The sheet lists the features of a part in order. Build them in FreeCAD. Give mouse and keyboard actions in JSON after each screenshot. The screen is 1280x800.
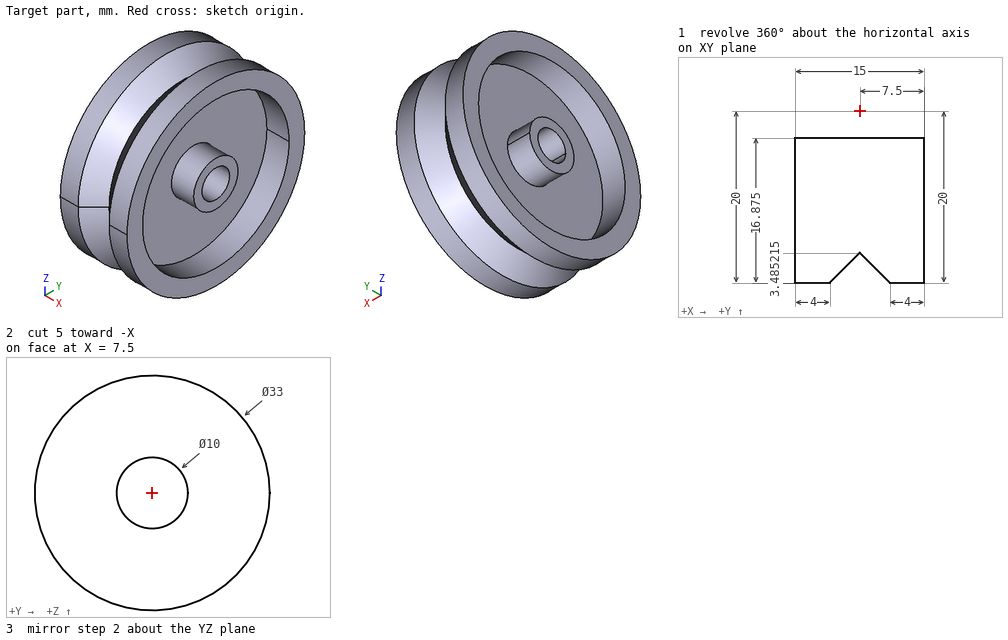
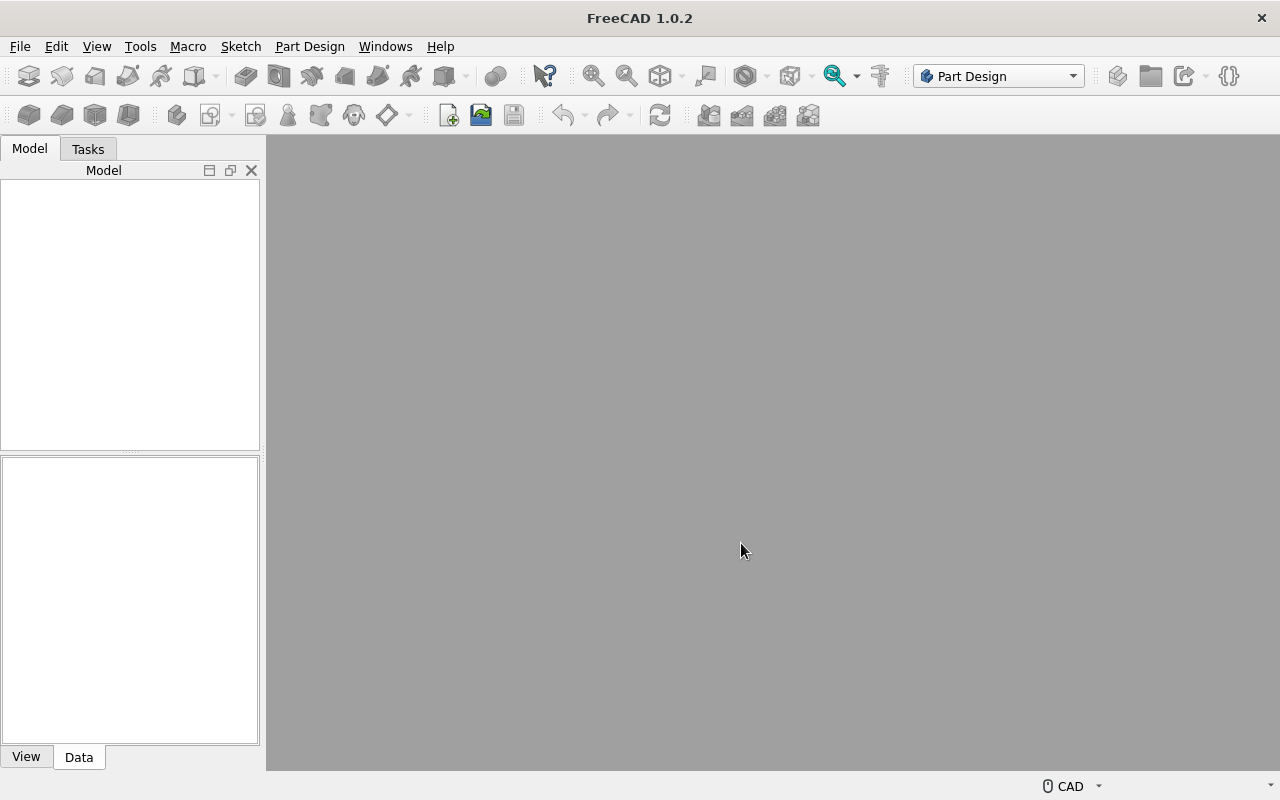
{"action": "left_click", "coordinate": [448, 116]}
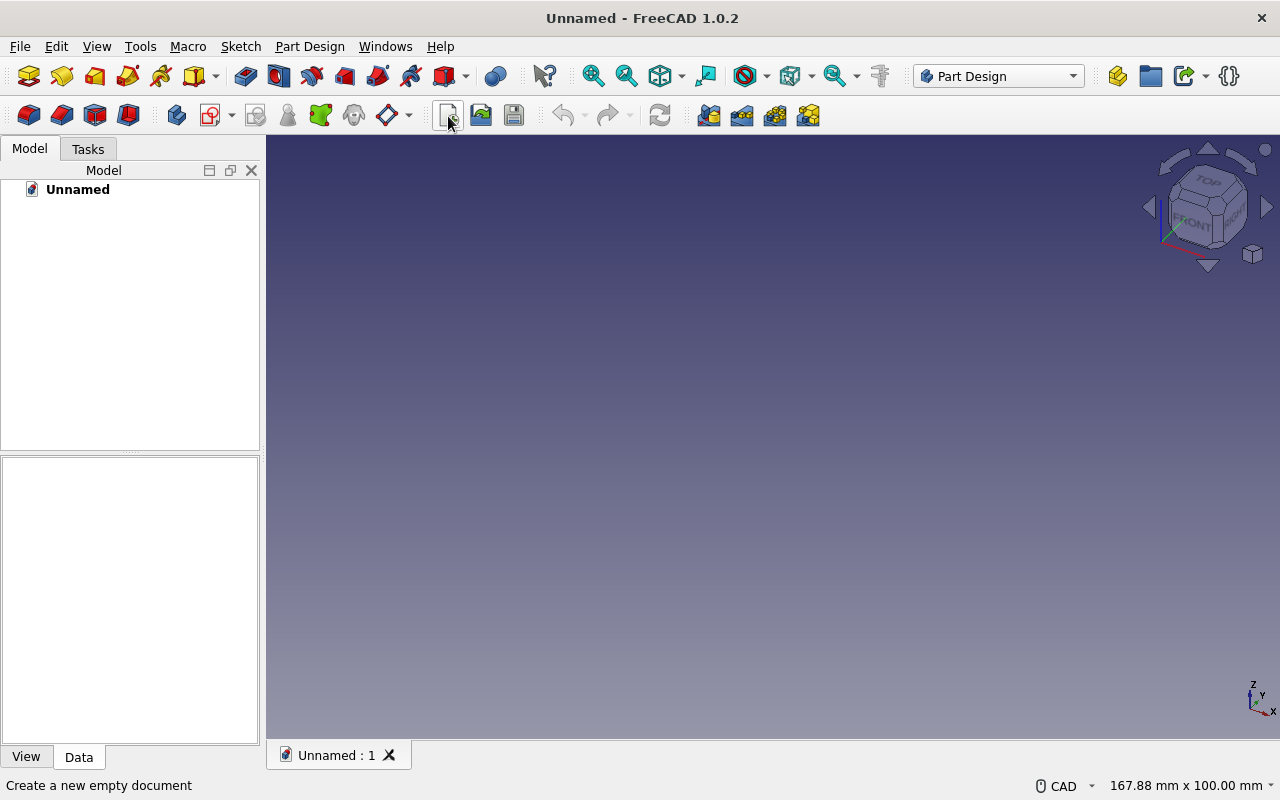
{"action": "left_click", "coordinate": [210, 116]}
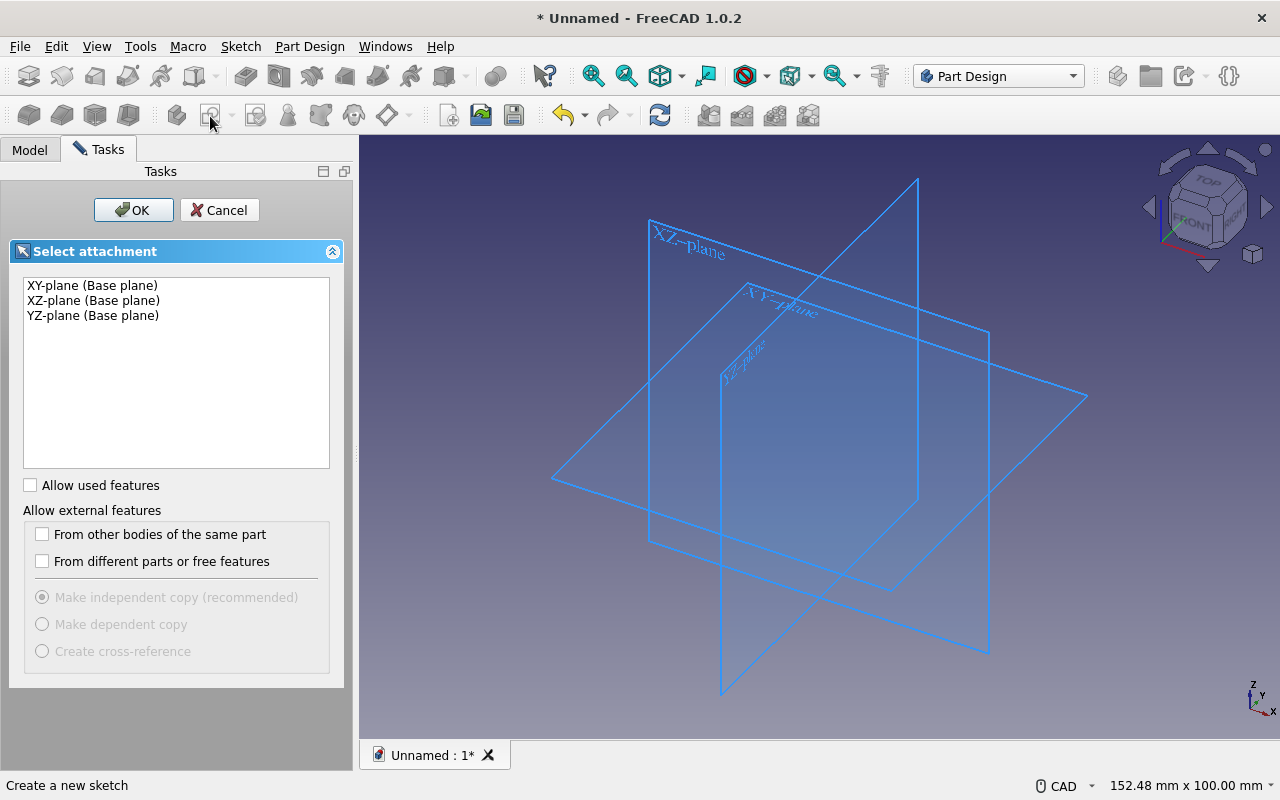
{"action": "left_click", "coordinate": [84, 286]}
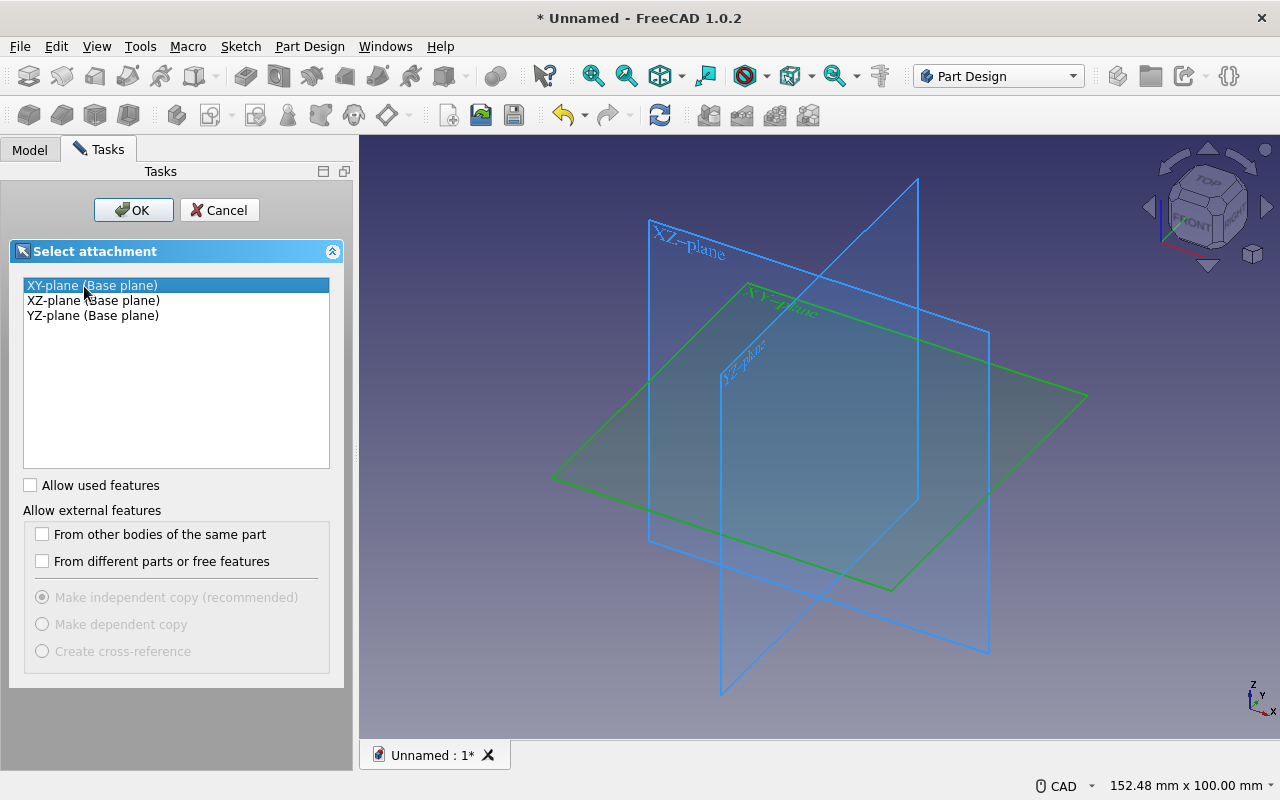
{"action": "left_click", "coordinate": [134, 210]}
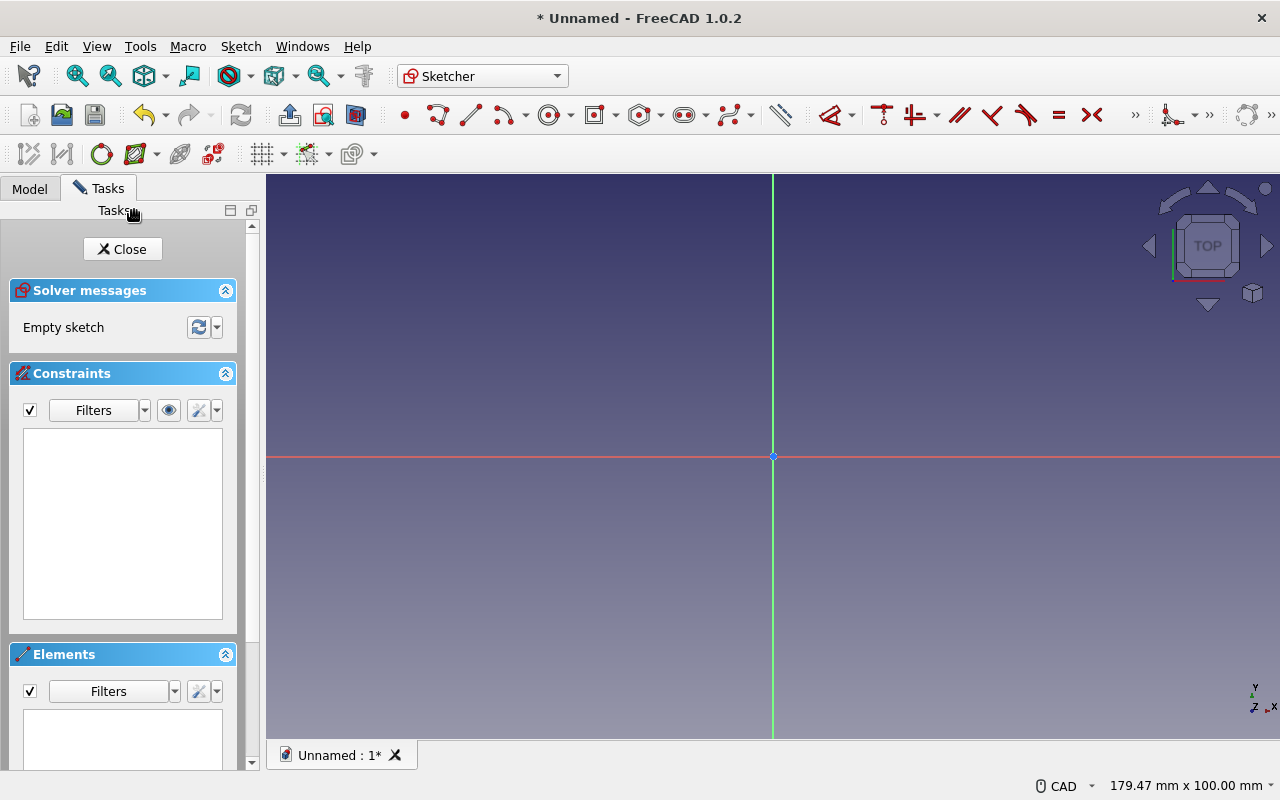
{"action": "scroll", "coordinate": [803, 537], "scroll_direction": "up", "scroll_amount": 6}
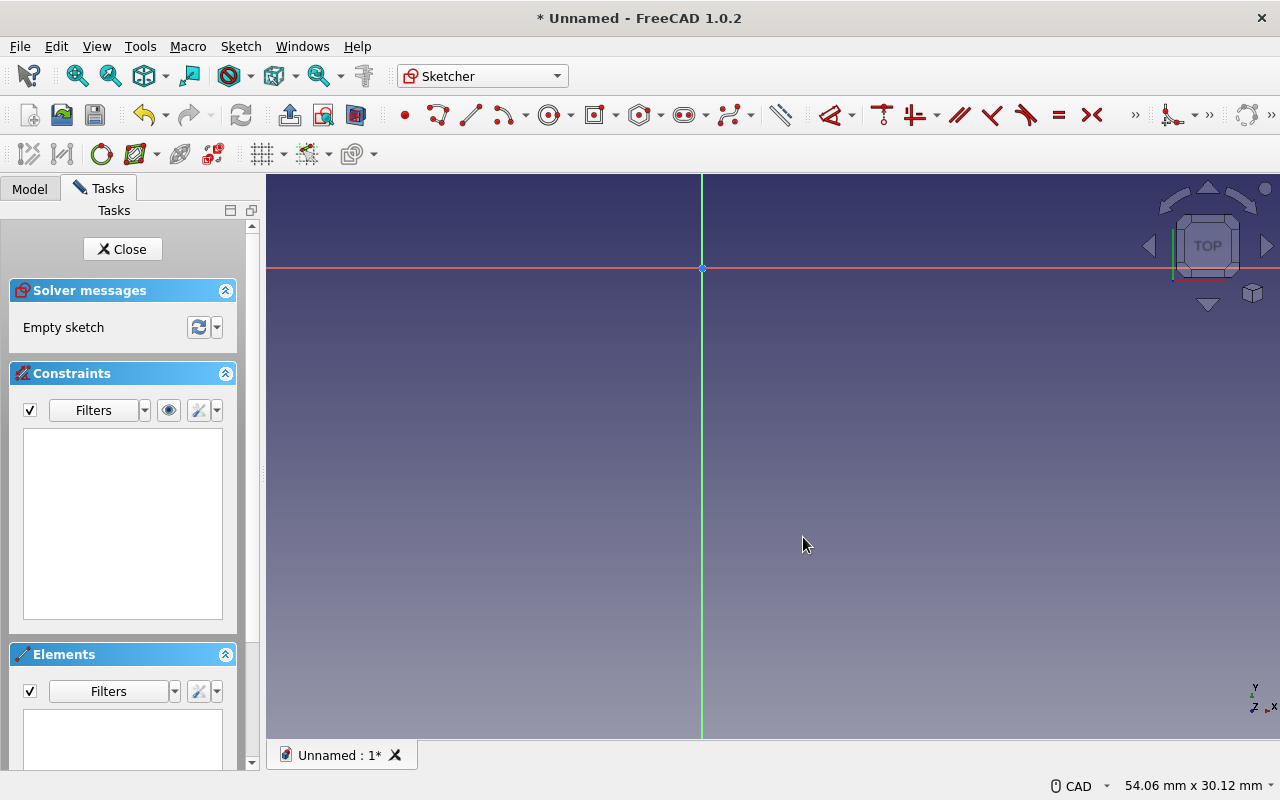
{"action": "left_click", "coordinate": [438, 116]}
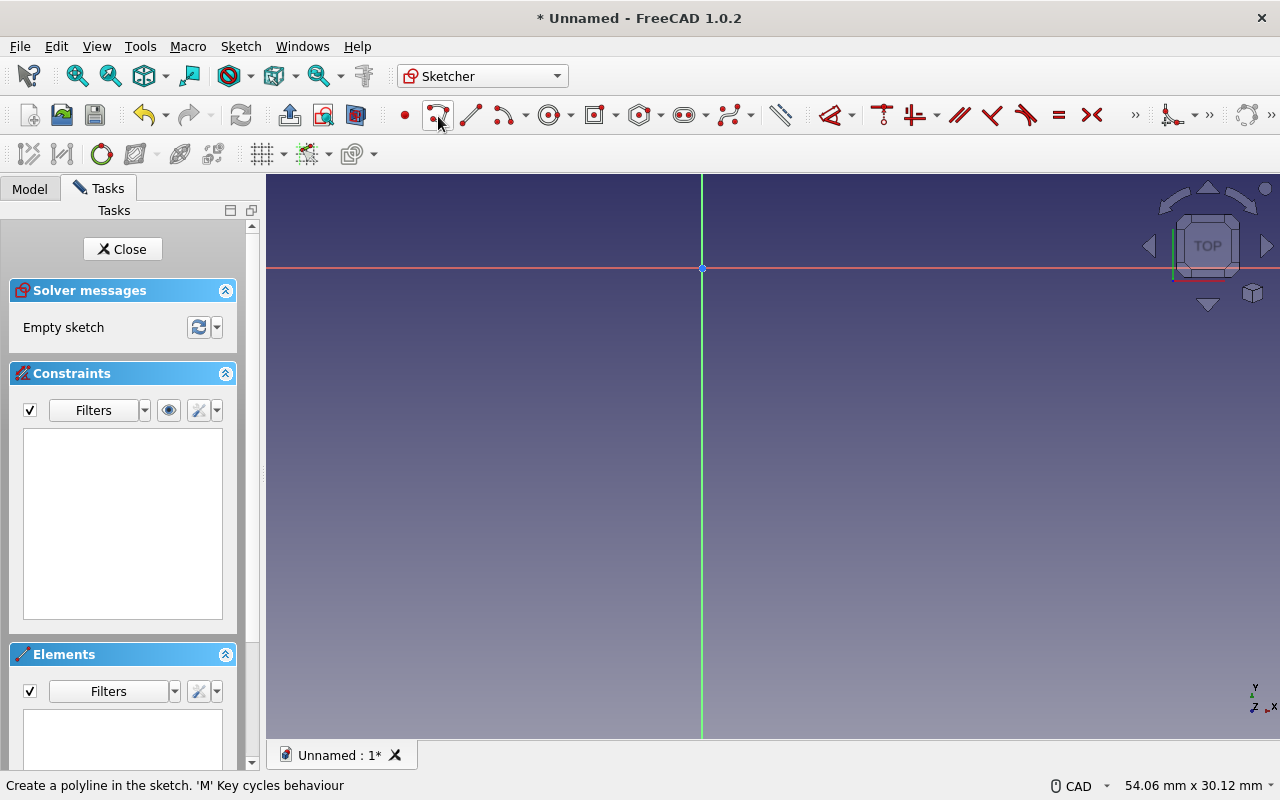
{"action": "left_click", "coordinate": [843, 327]}
{"action": "left_click", "coordinate": [561, 327]}
{"action": "left_click", "coordinate": [561, 643]}
{"action": "left_click", "coordinate": [637, 643]}
{"action": "left_click", "coordinate": [702, 578]}
{"action": "left_click", "coordinate": [768, 643]}
{"action": "left_click", "coordinate": [843, 643]}
{"action": "left_click", "coordinate": [843, 328]}
{"action": "key", "text": "Escape"}
{"action": "key", "text": "Escape"}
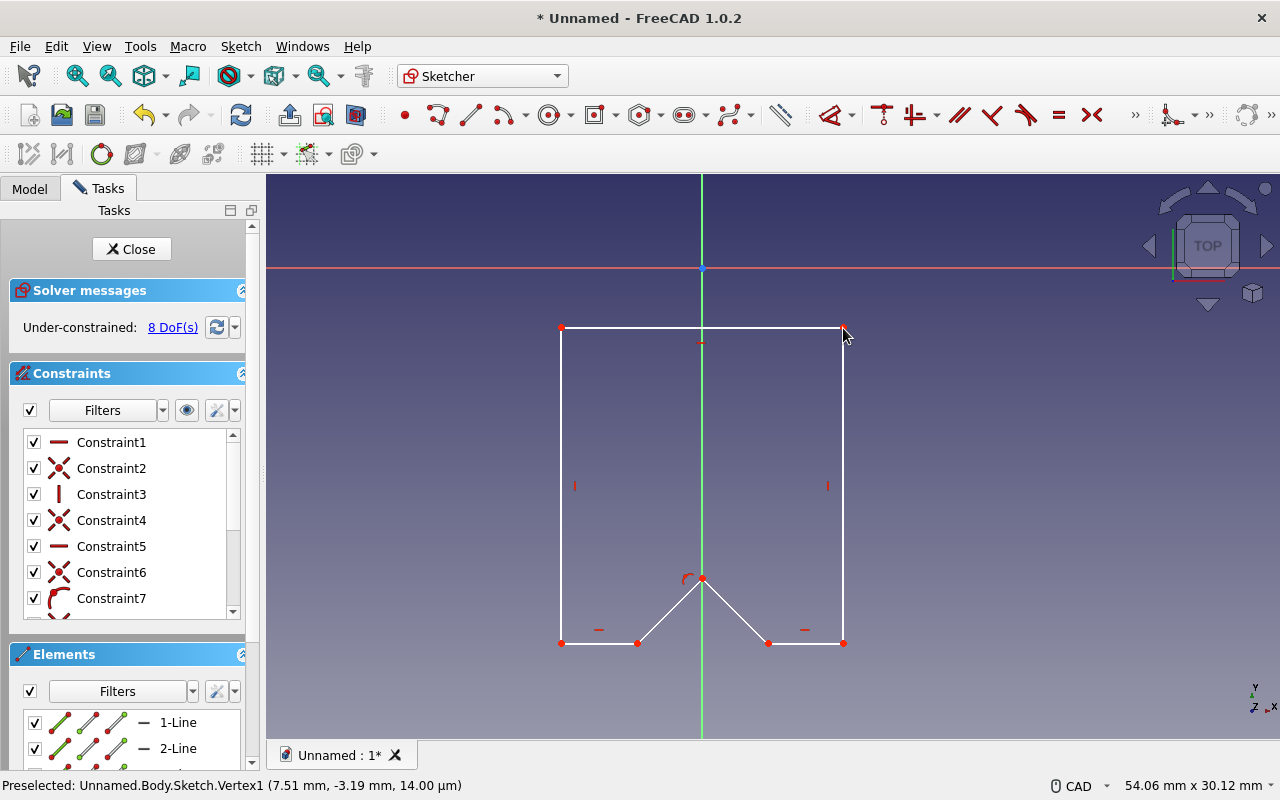
{"action": "left_click", "coordinate": [830, 116]}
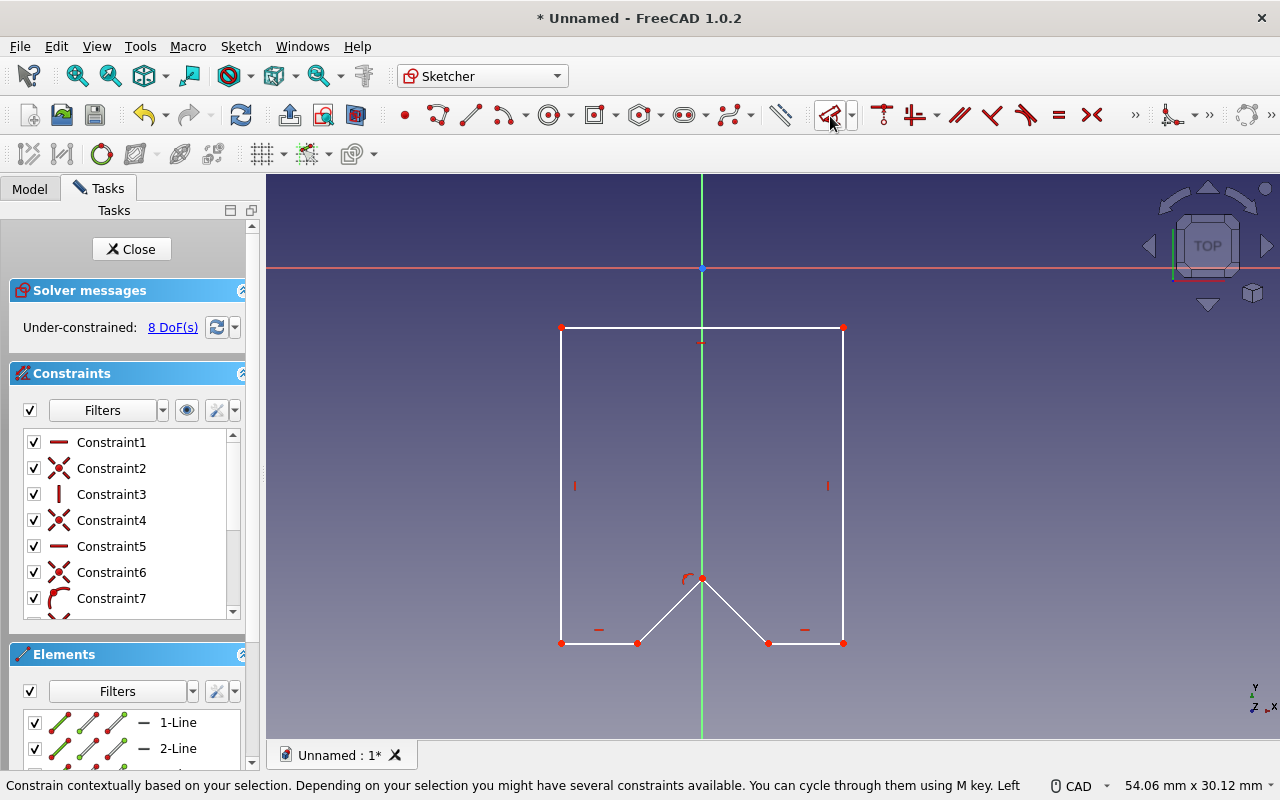
{"action": "left_click", "coordinate": [584, 644]}
{"action": "left_click", "coordinate": [599, 678]}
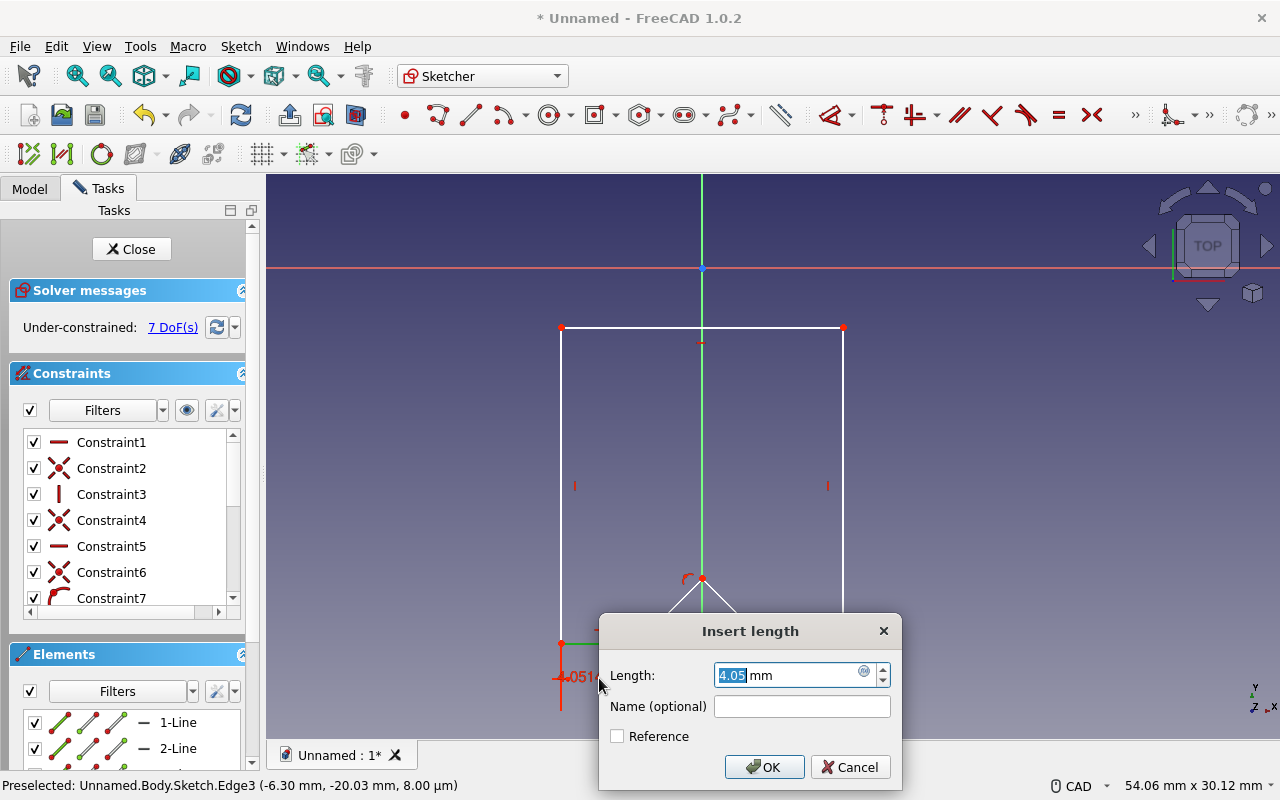
{"action": "type", "text": "4"}
{"action": "key", "text": "Return"}